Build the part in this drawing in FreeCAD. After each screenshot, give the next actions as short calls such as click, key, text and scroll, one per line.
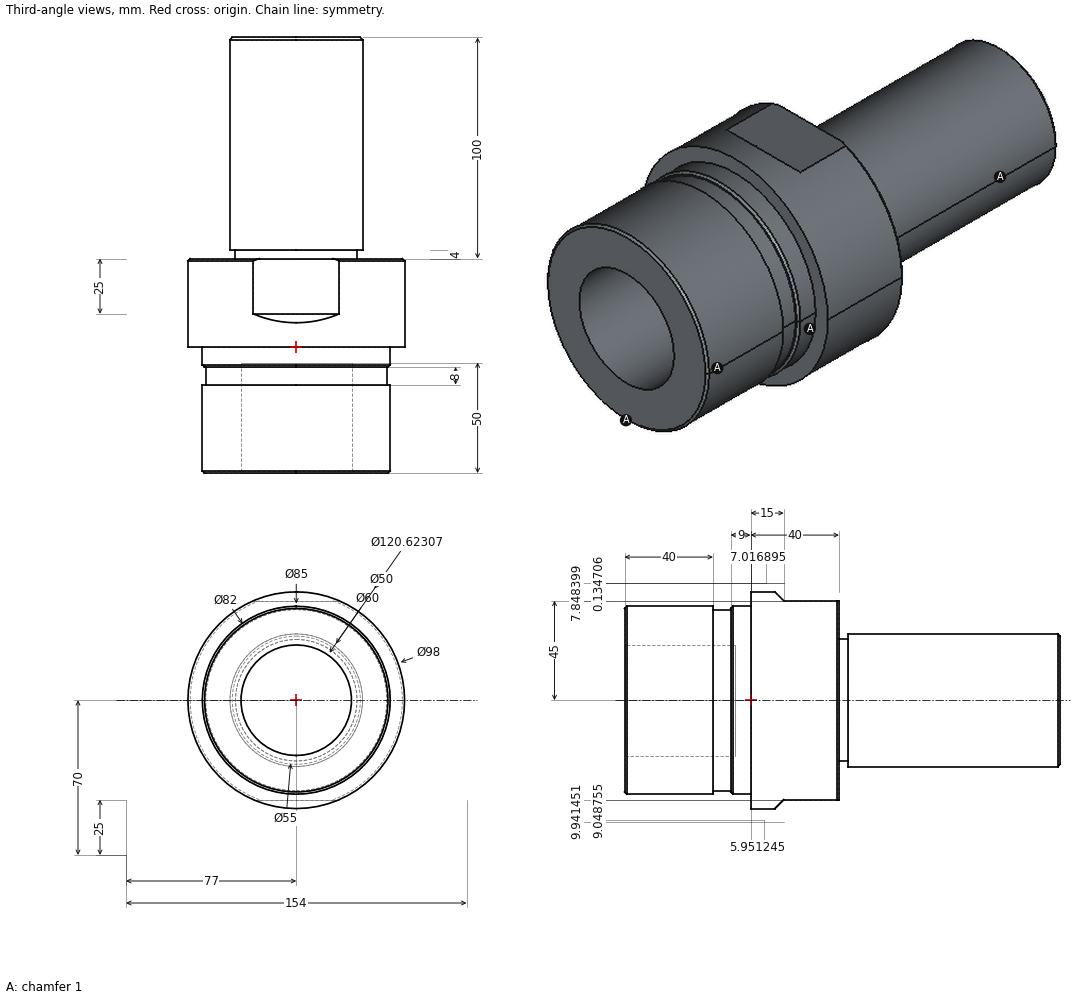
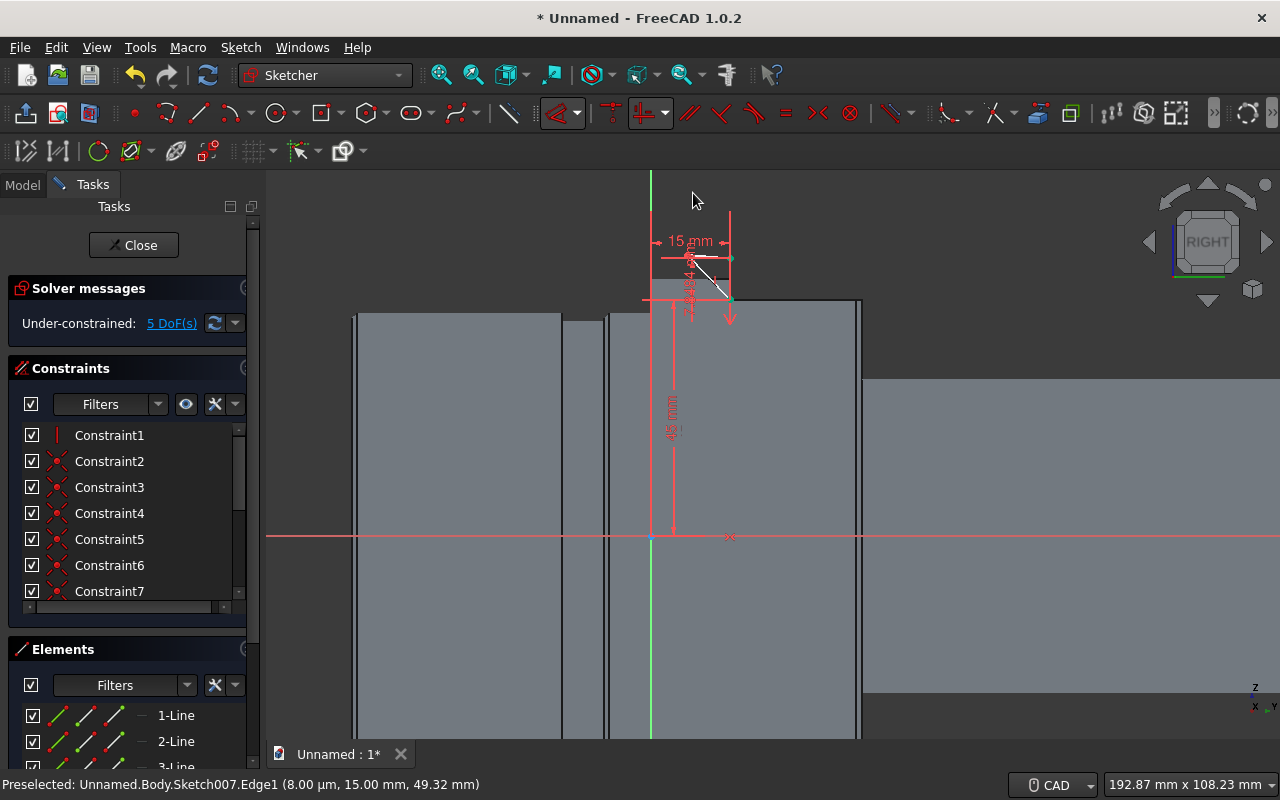
scroll(733, 278, down, 2)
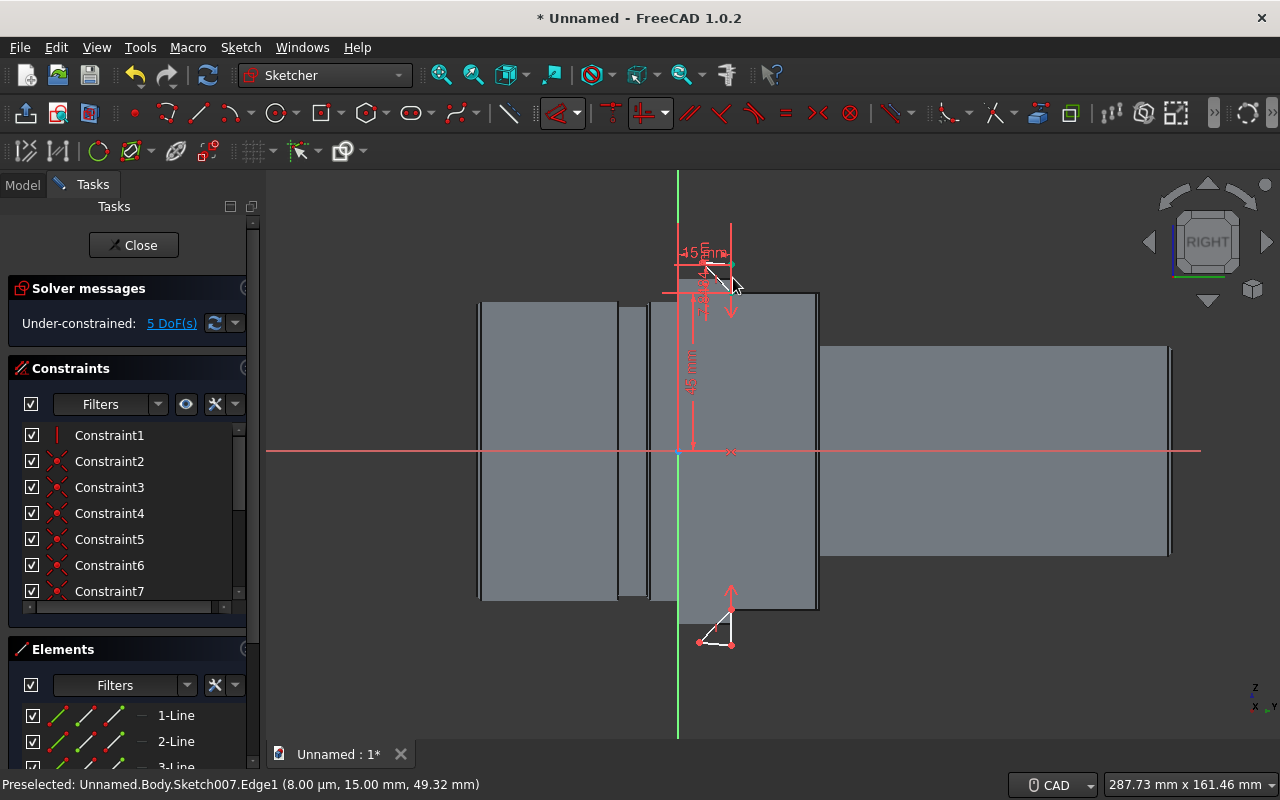
scroll(731, 635, up, 2)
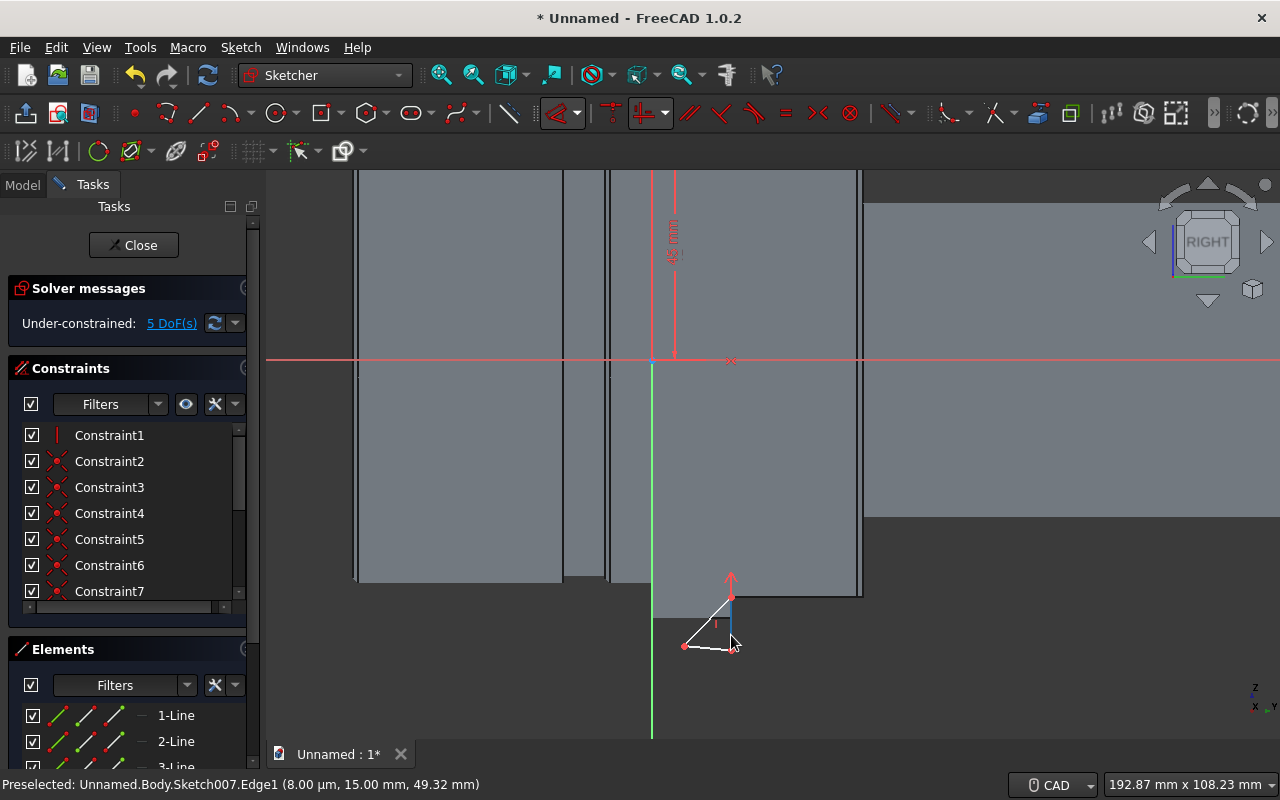
click(731, 634)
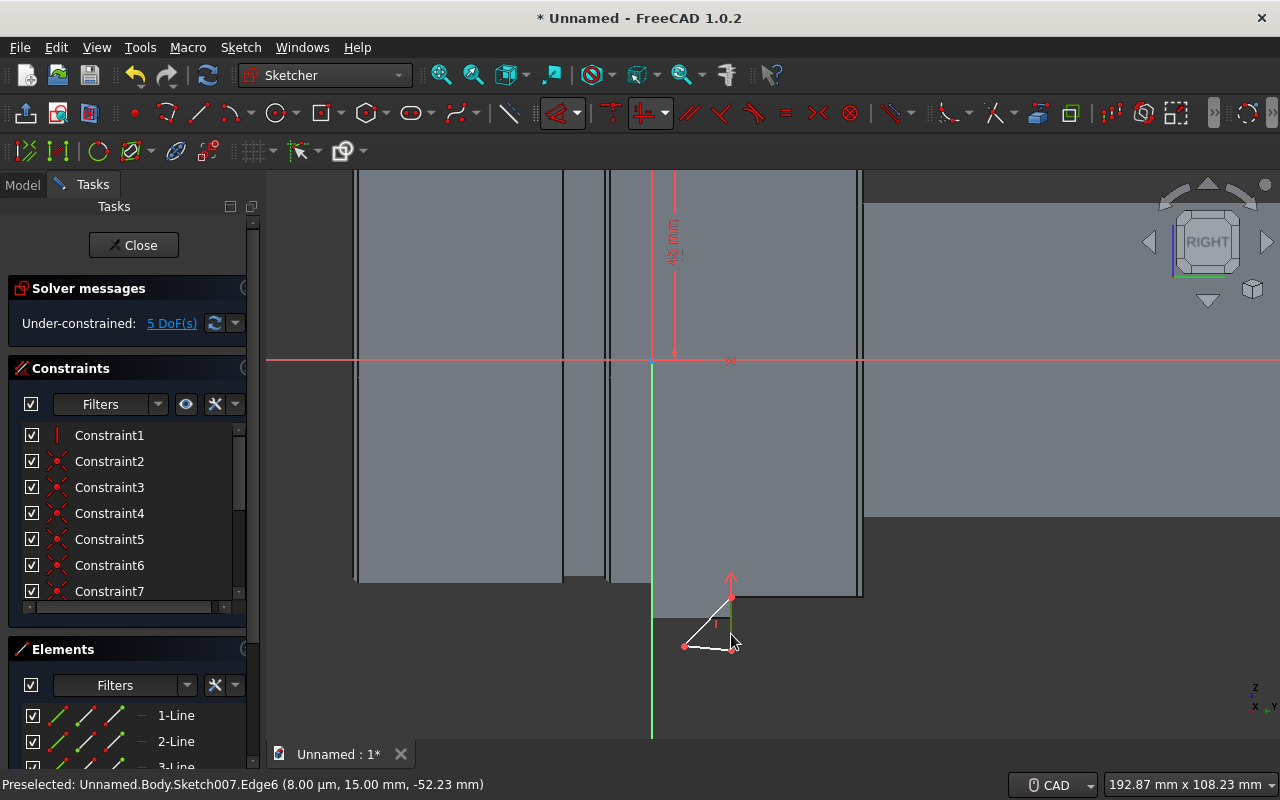
key(i)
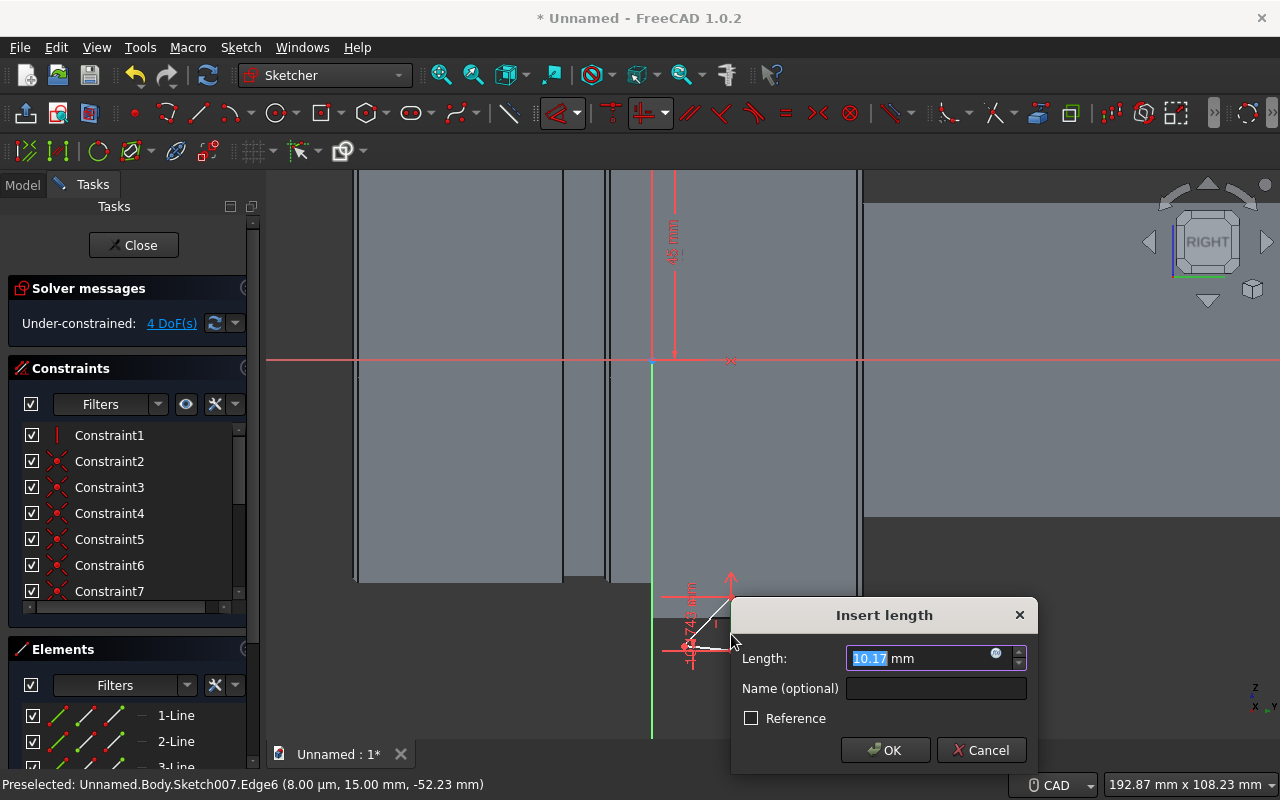
text(9.941451)
key(Return)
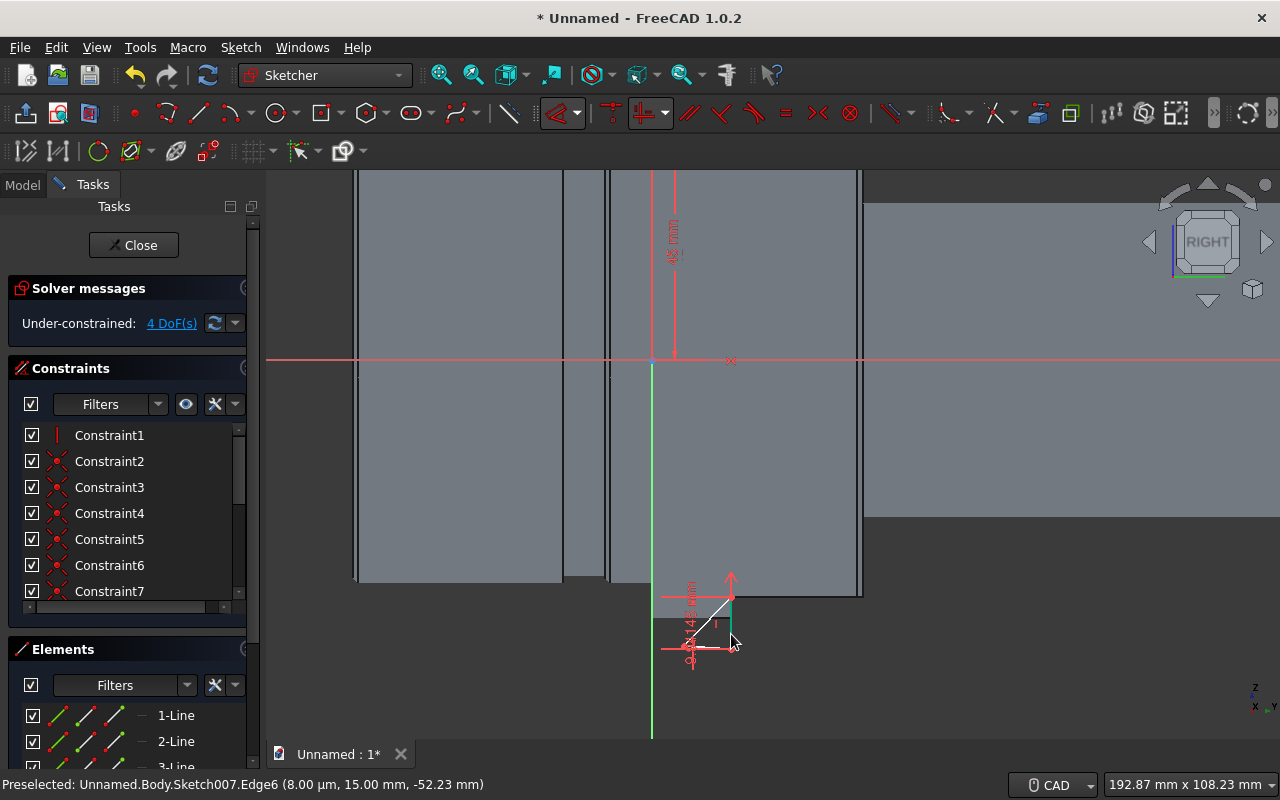
scroll(731, 635, down, 2)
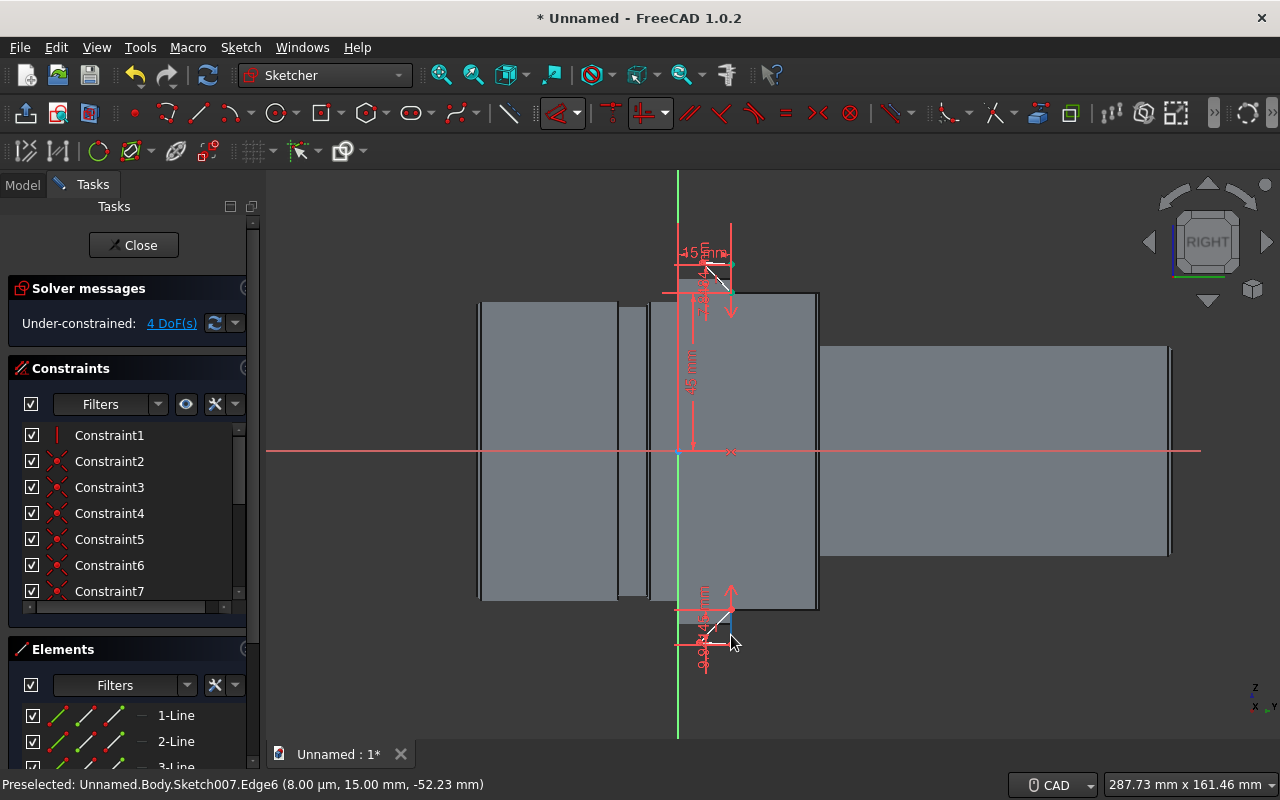
scroll(703, 263, up, 3)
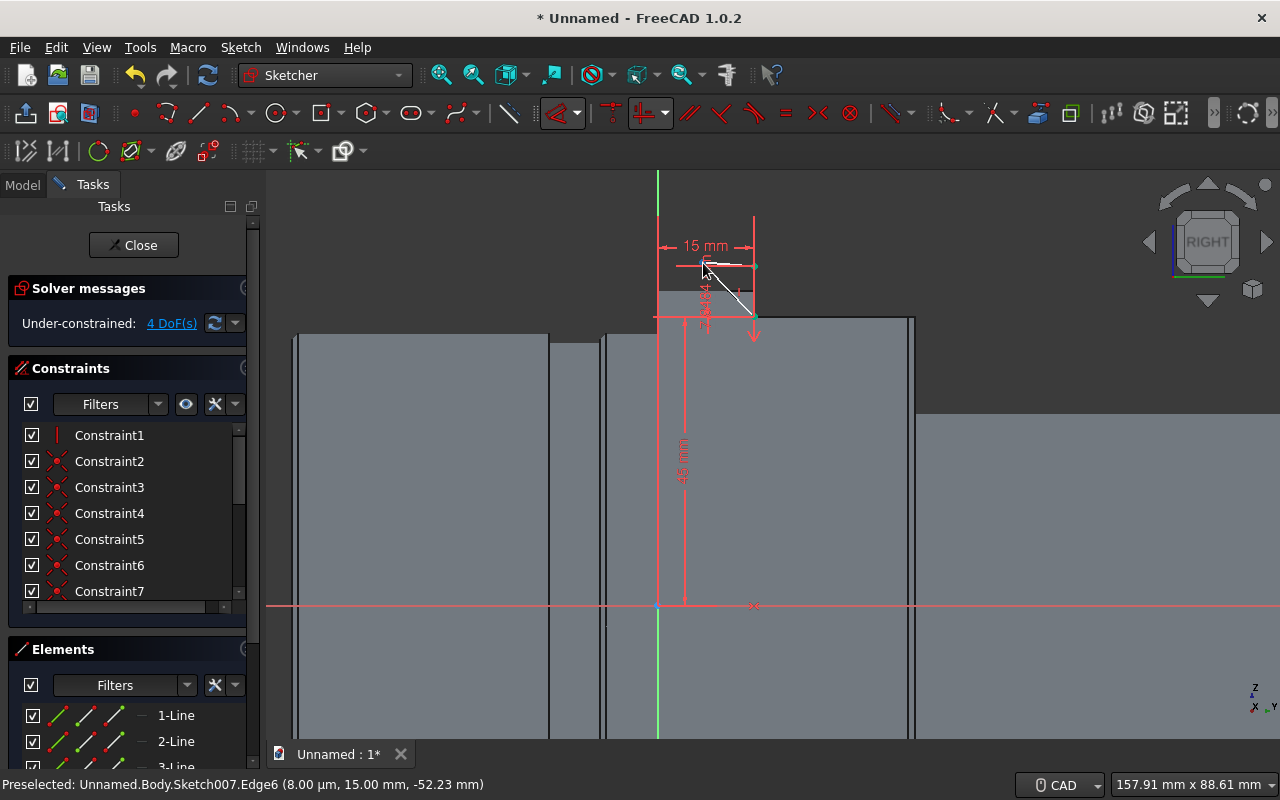
click(702, 262)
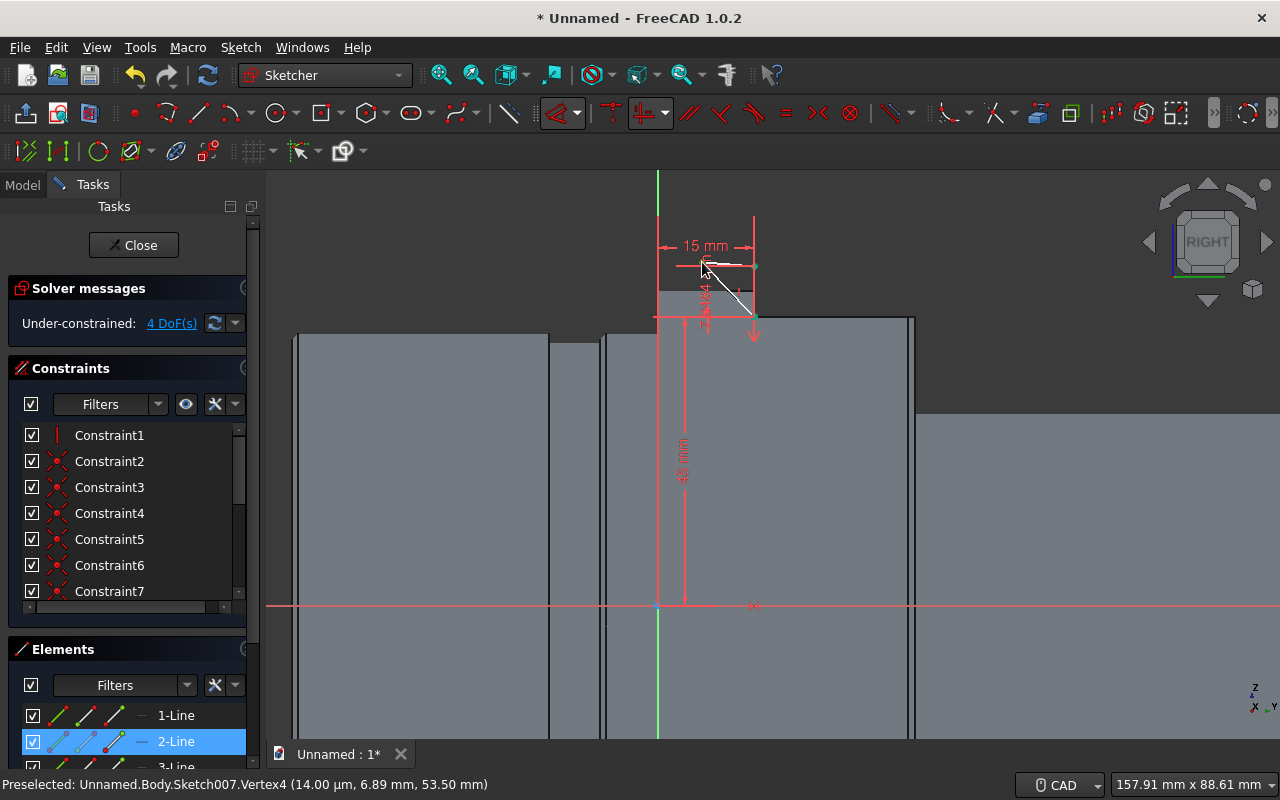
click(580, 114)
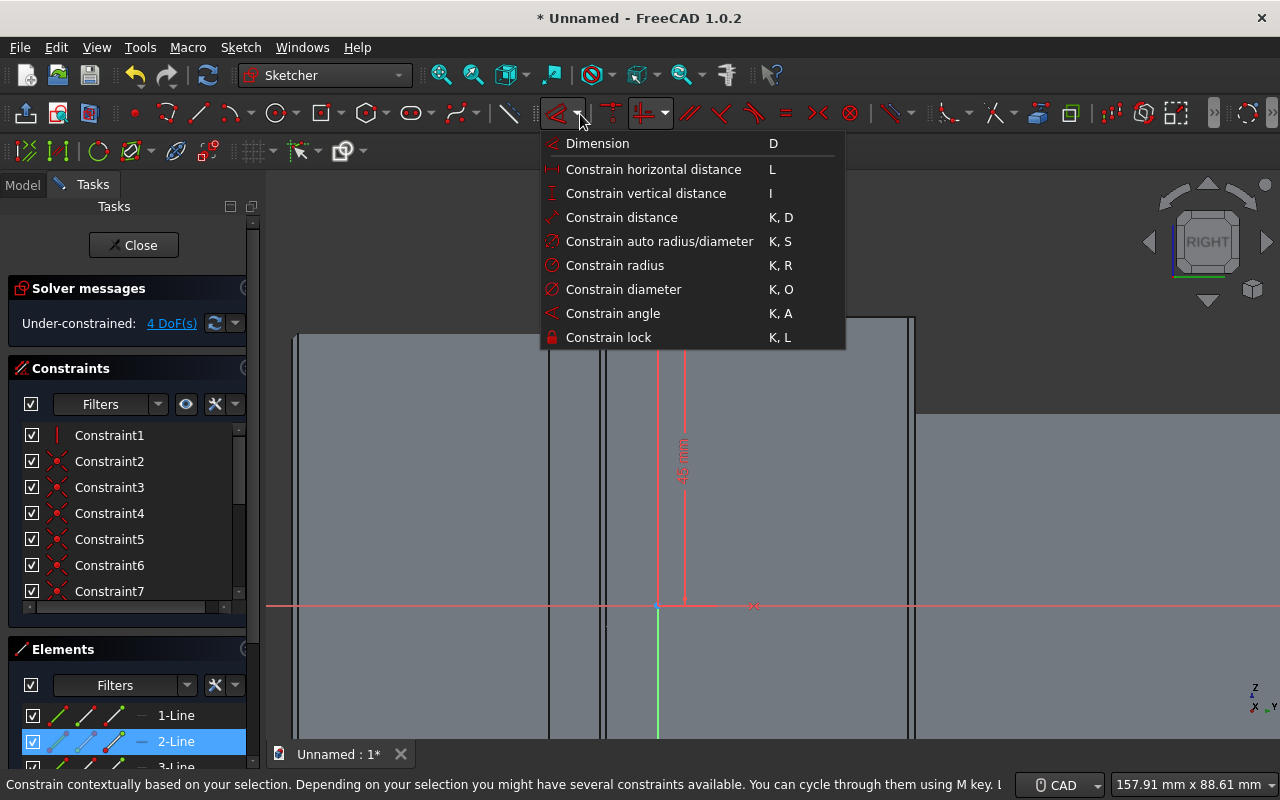
click(693, 169)